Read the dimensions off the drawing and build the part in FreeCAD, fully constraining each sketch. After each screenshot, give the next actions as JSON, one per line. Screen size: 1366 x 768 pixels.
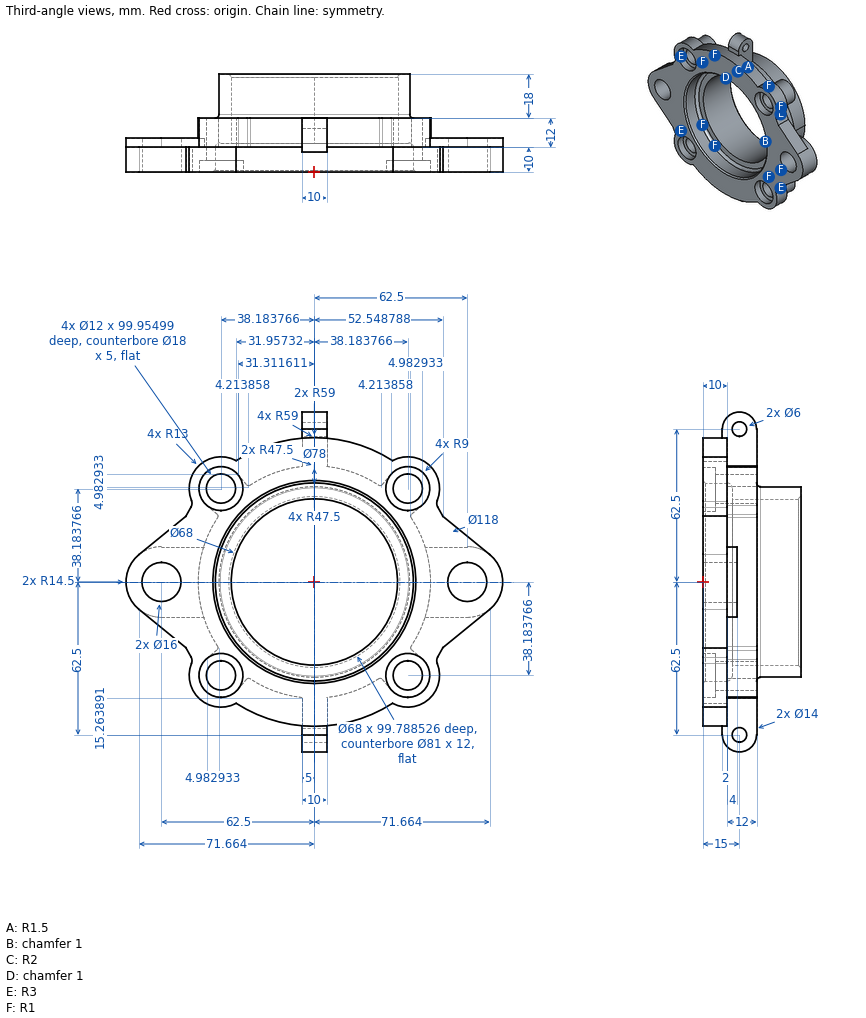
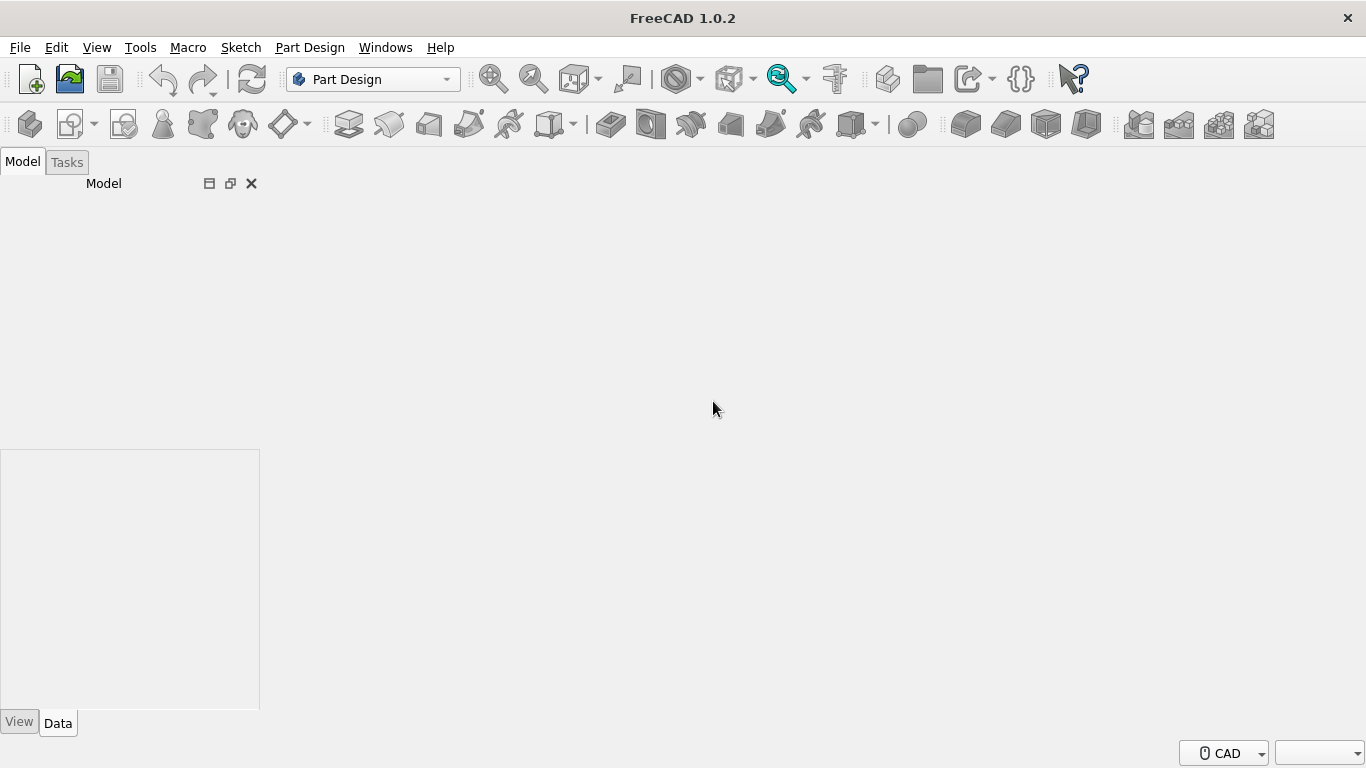
{"action": "left_click", "coordinate": [30, 80]}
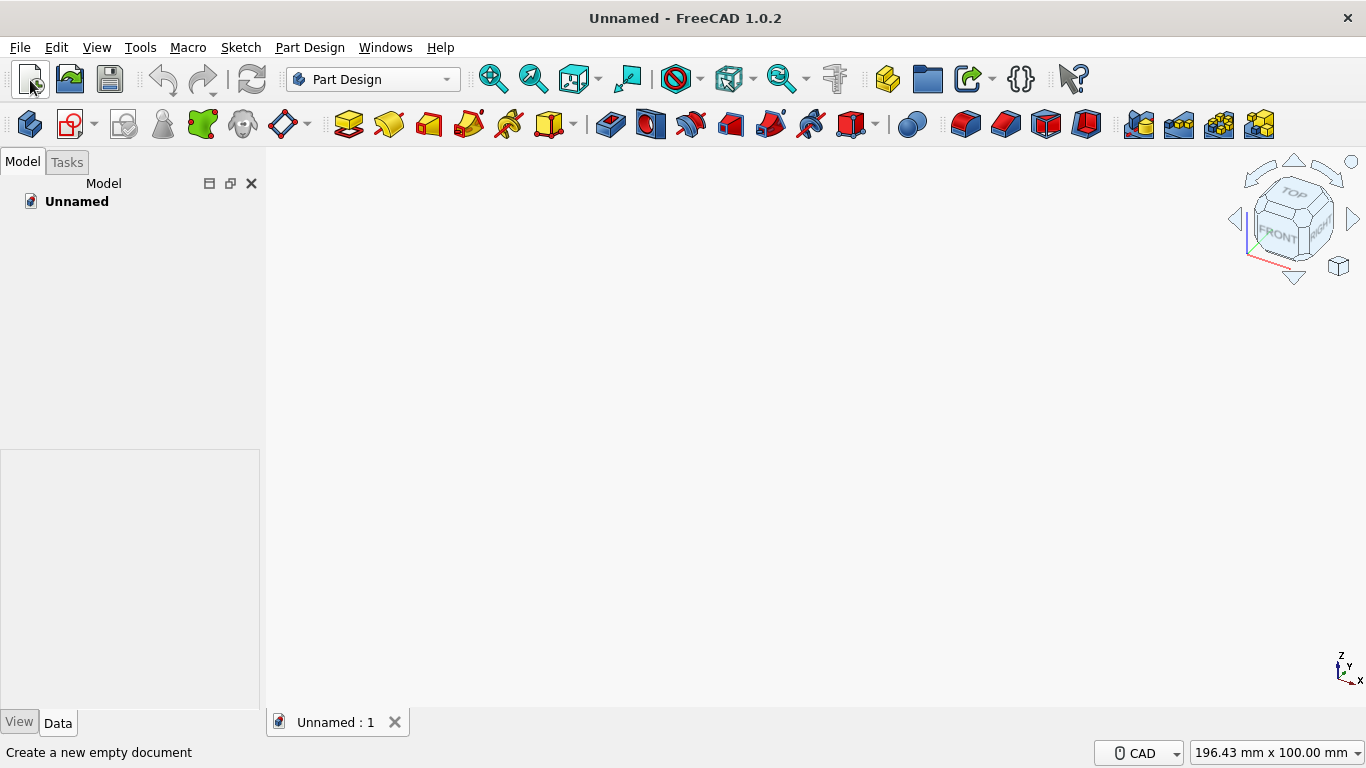
{"action": "left_click", "coordinate": [70, 124]}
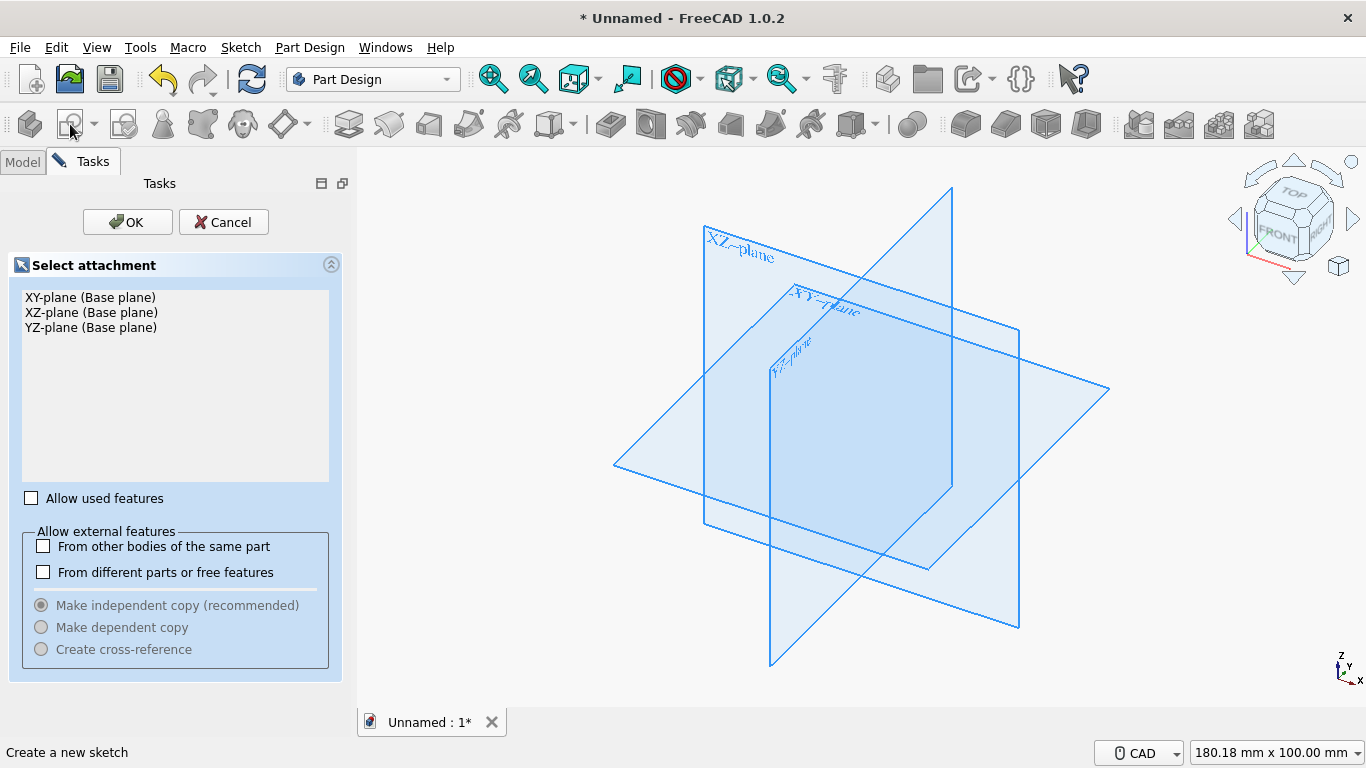
{"action": "left_click", "coordinate": [82, 312]}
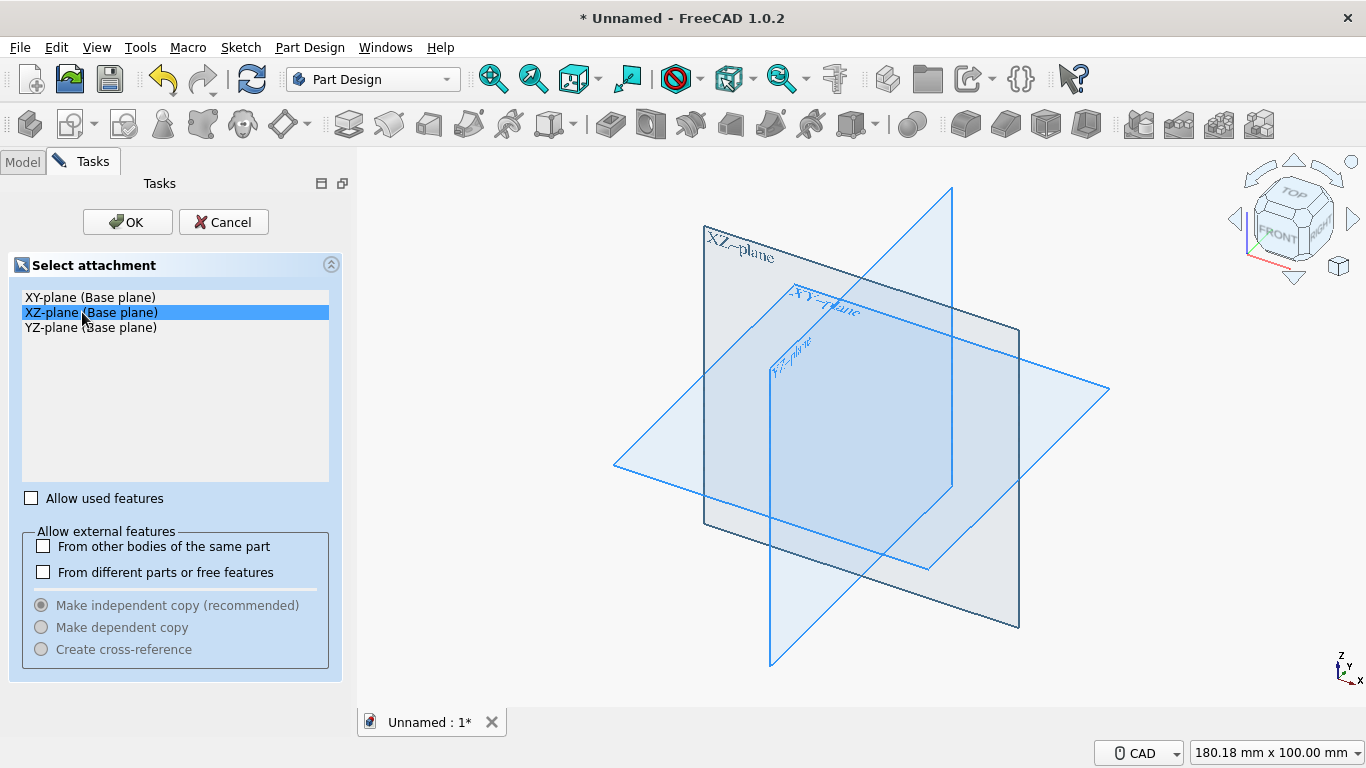
{"action": "left_click", "coordinate": [128, 222]}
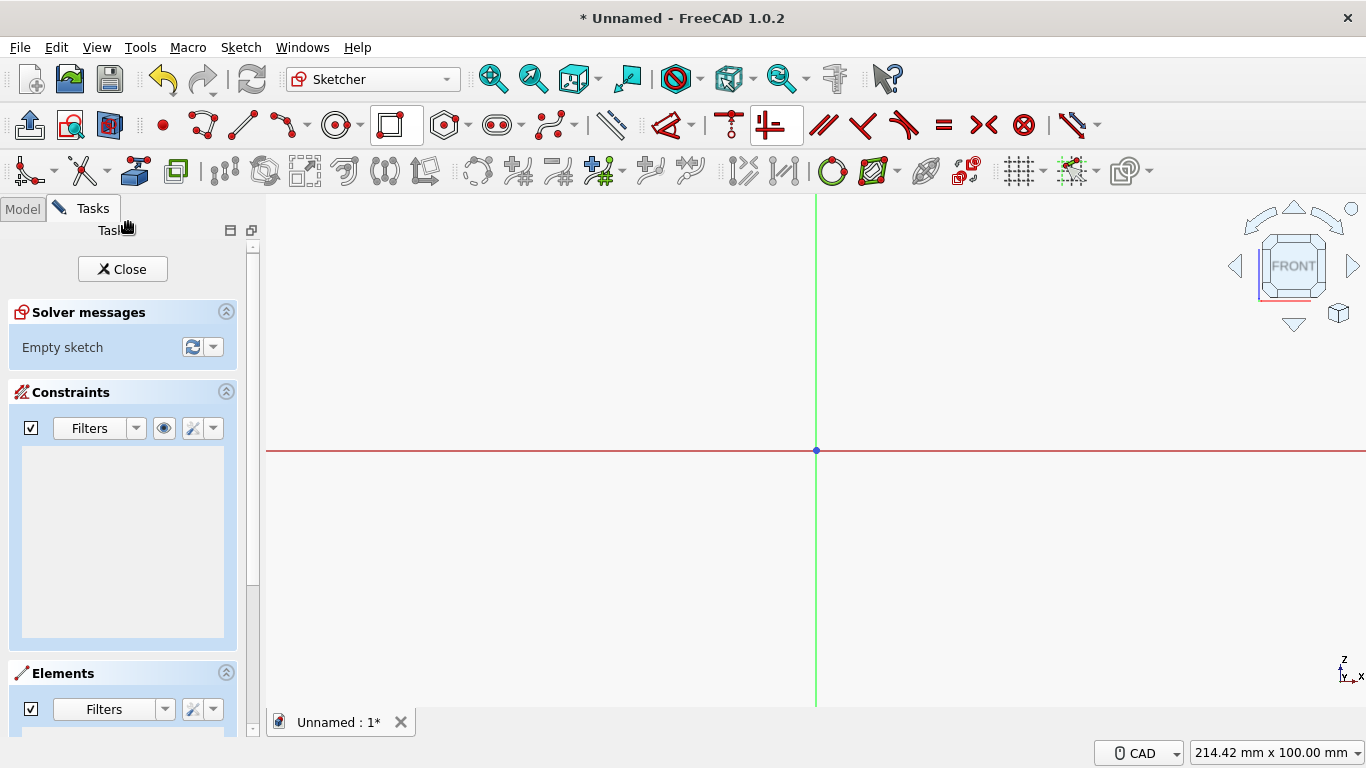
{"action": "scroll", "coordinate": [664, 451], "scroll_direction": "down", "scroll_amount": 3}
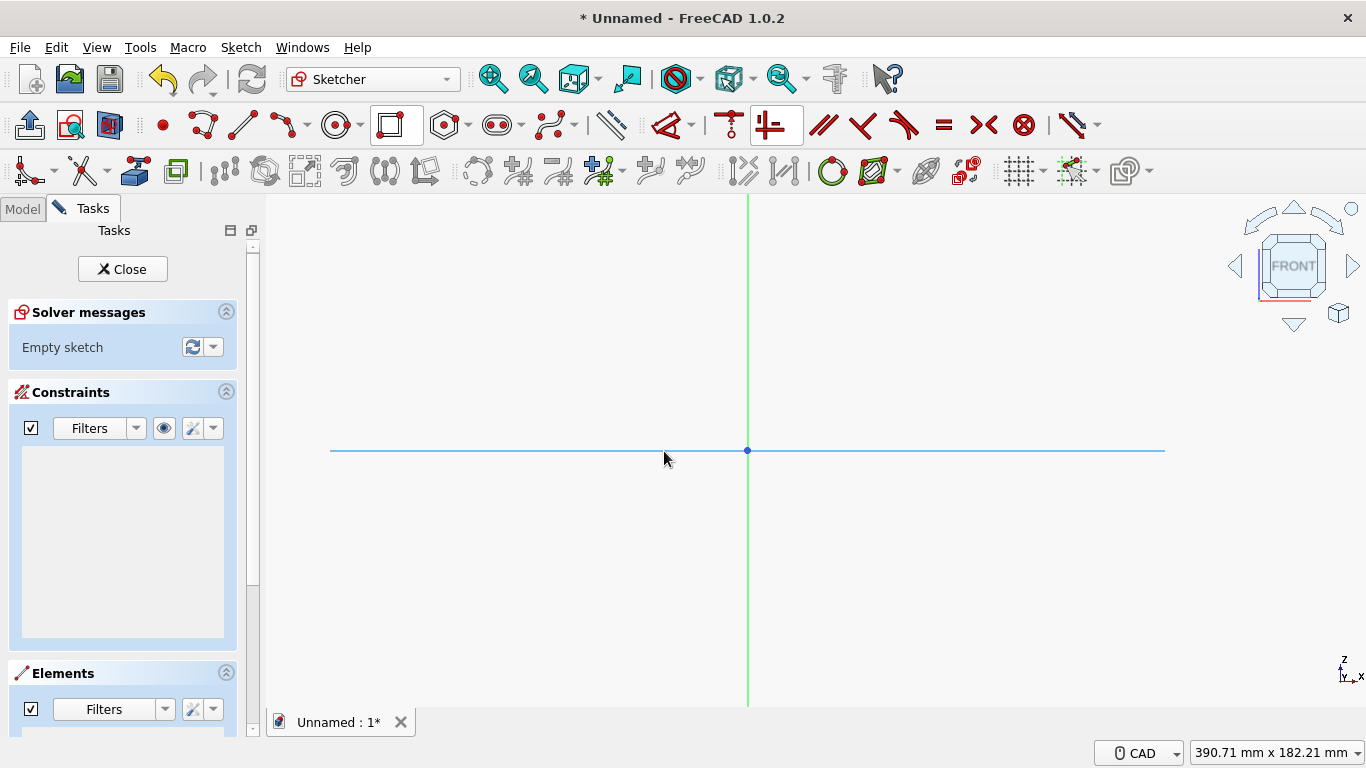
{"action": "left_click", "coordinate": [336, 126]}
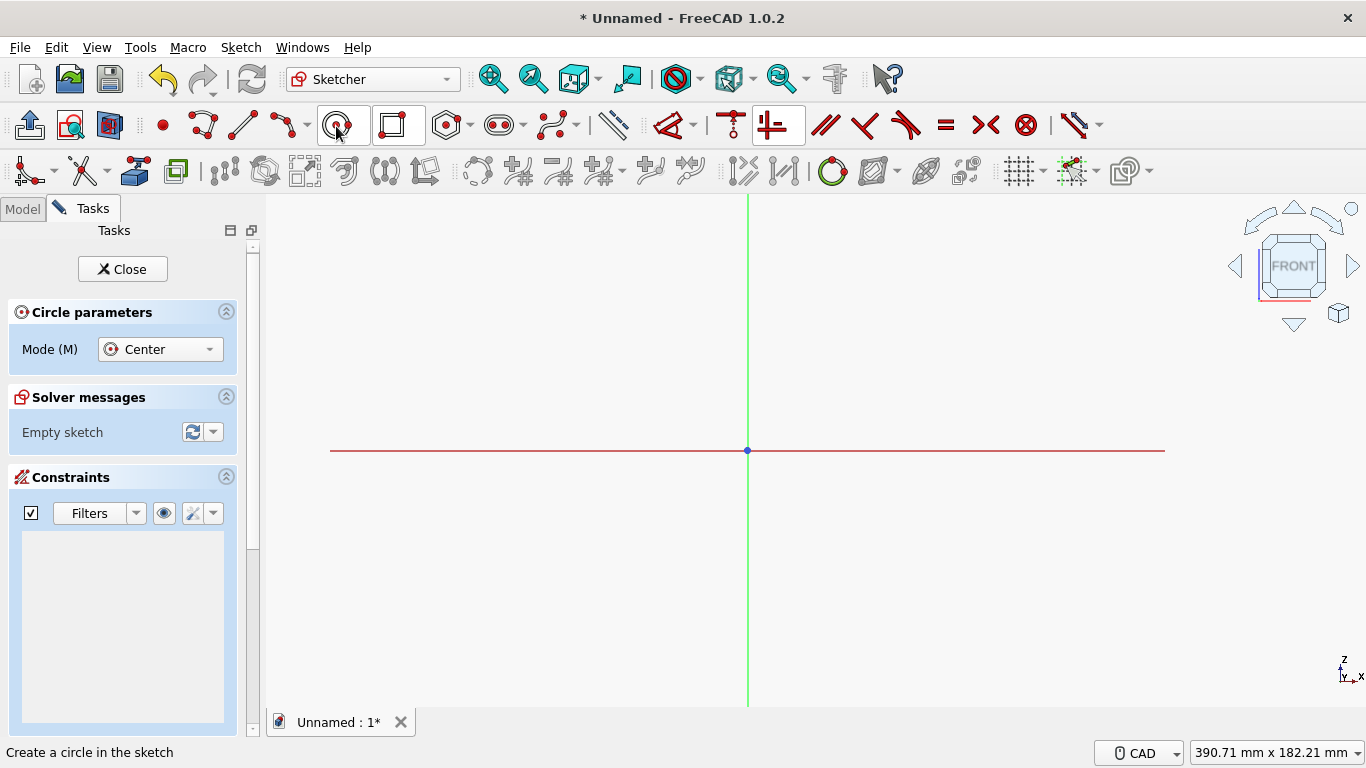
{"action": "left_click", "coordinate": [748, 451]}
{"action": "left_click", "coordinate": [865, 333]}
{"action": "key", "text": "Escape"}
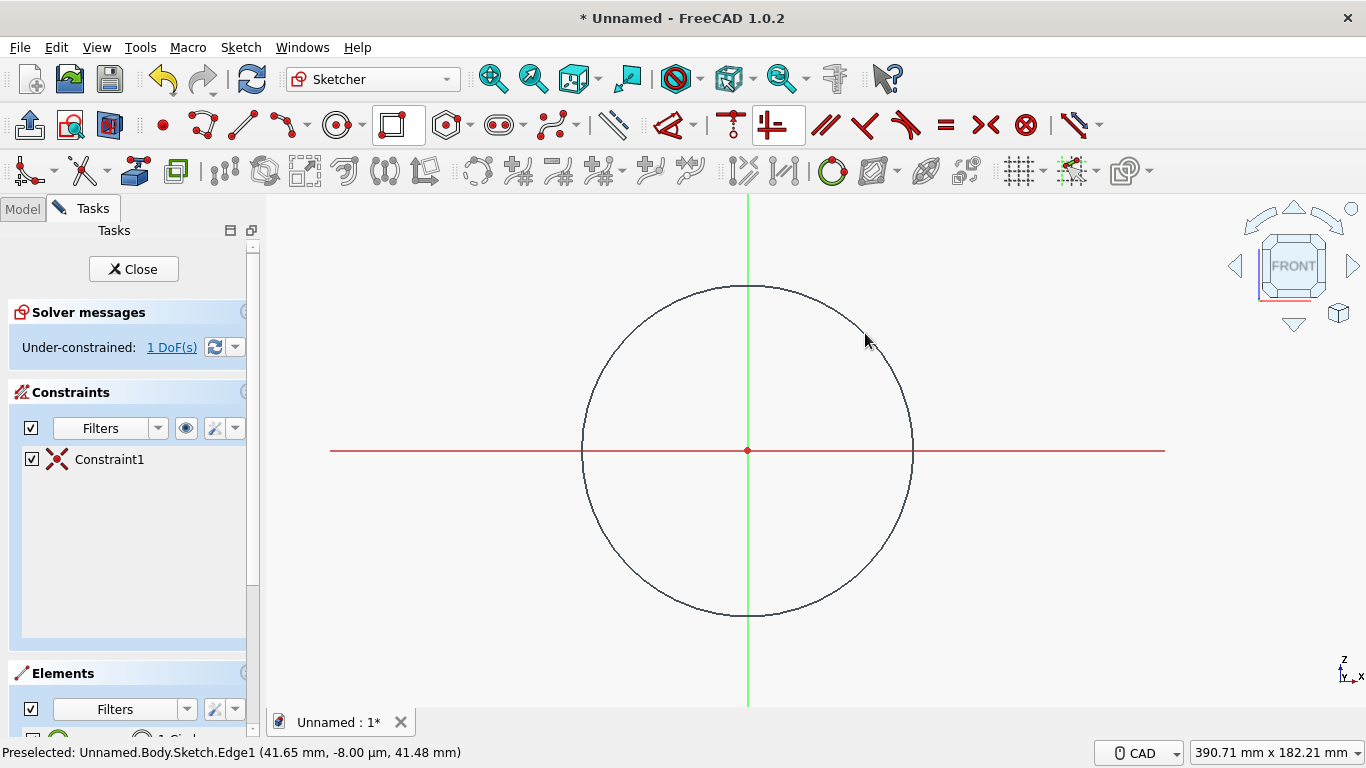
{"action": "left_click", "coordinate": [864, 333]}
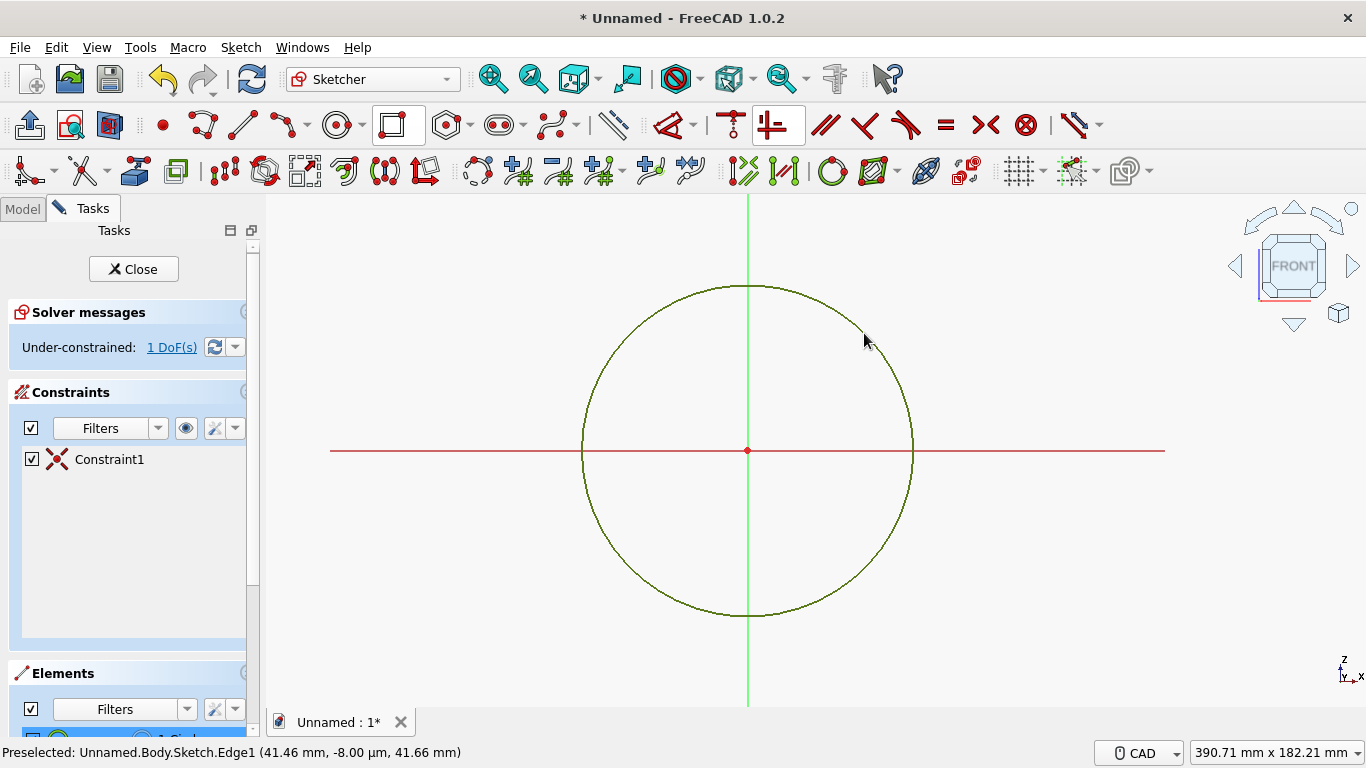
{"action": "left_click", "coordinate": [696, 126]}